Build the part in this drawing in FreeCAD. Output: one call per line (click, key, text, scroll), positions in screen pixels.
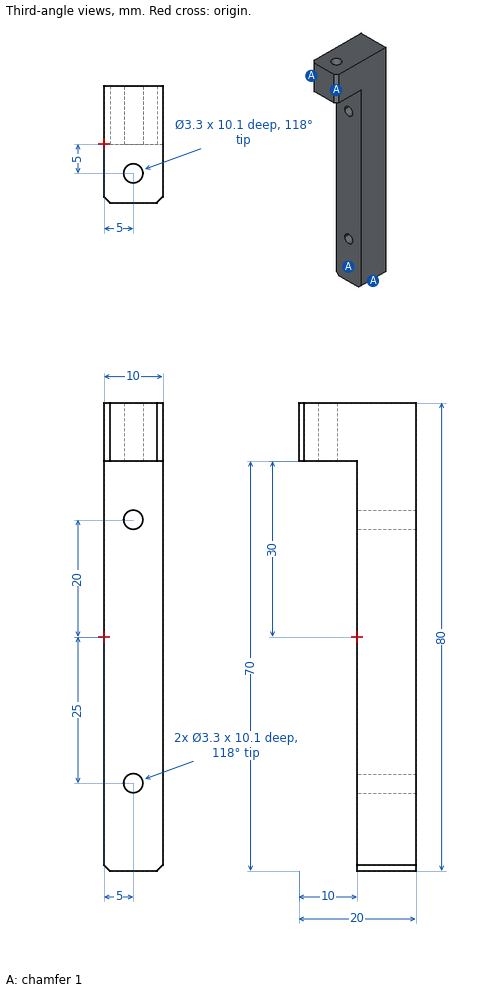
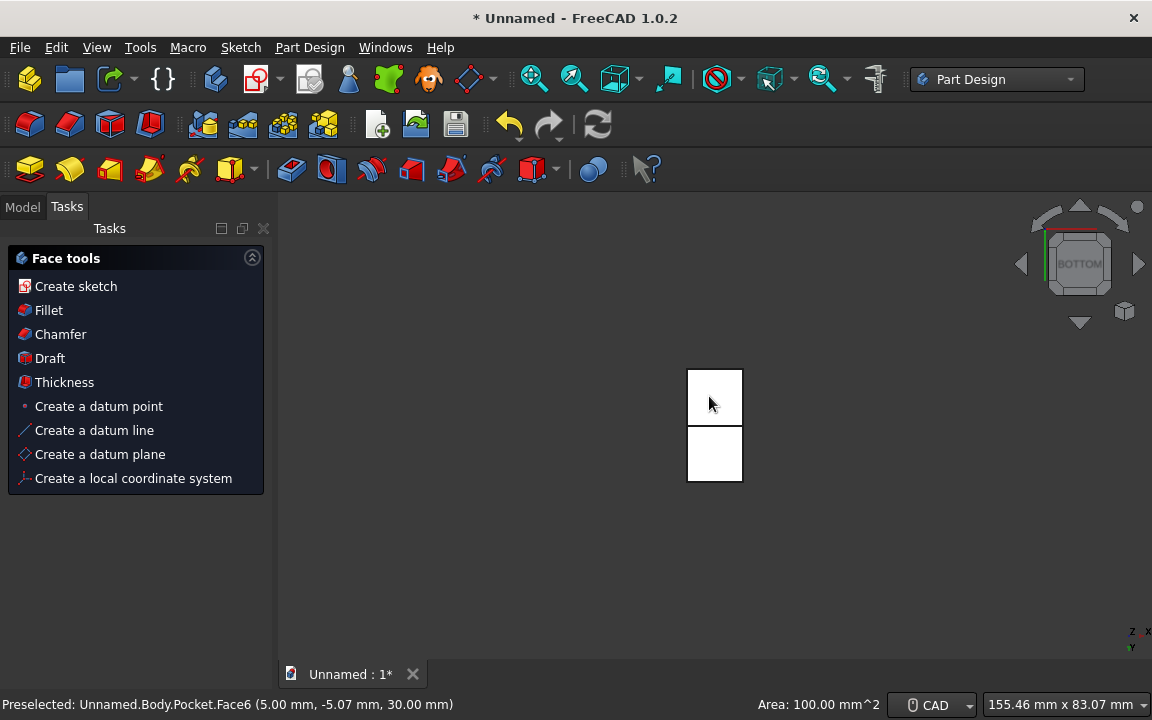
click(256, 80)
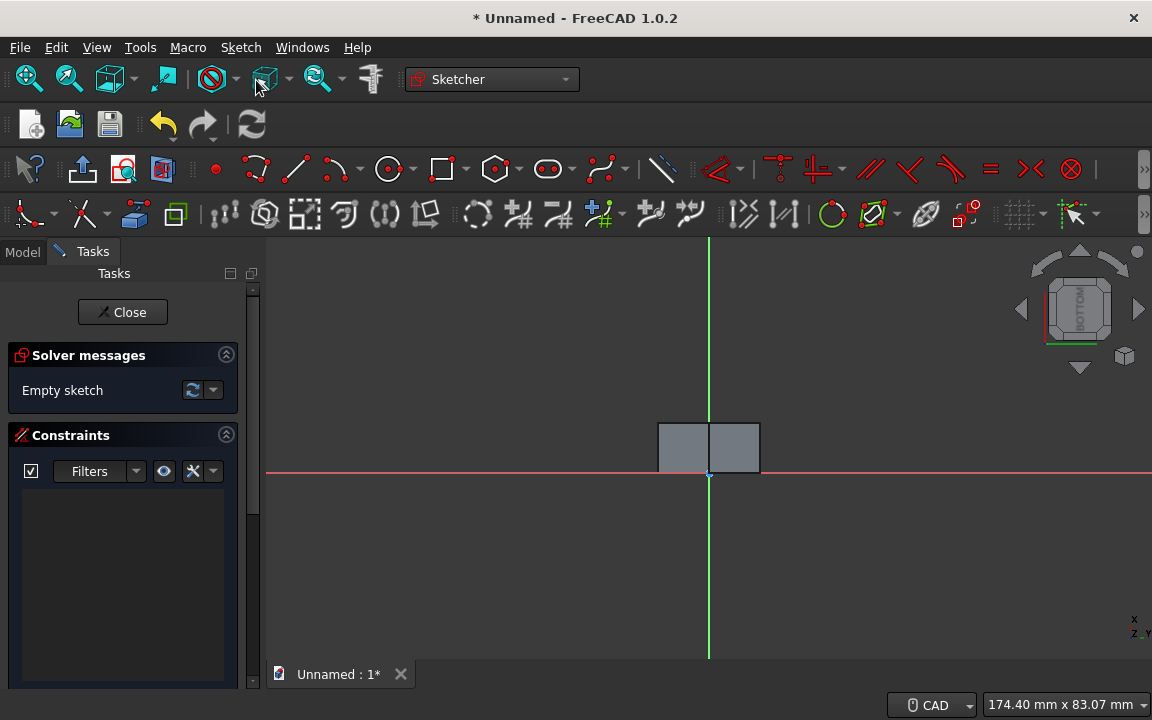
click(164, 170)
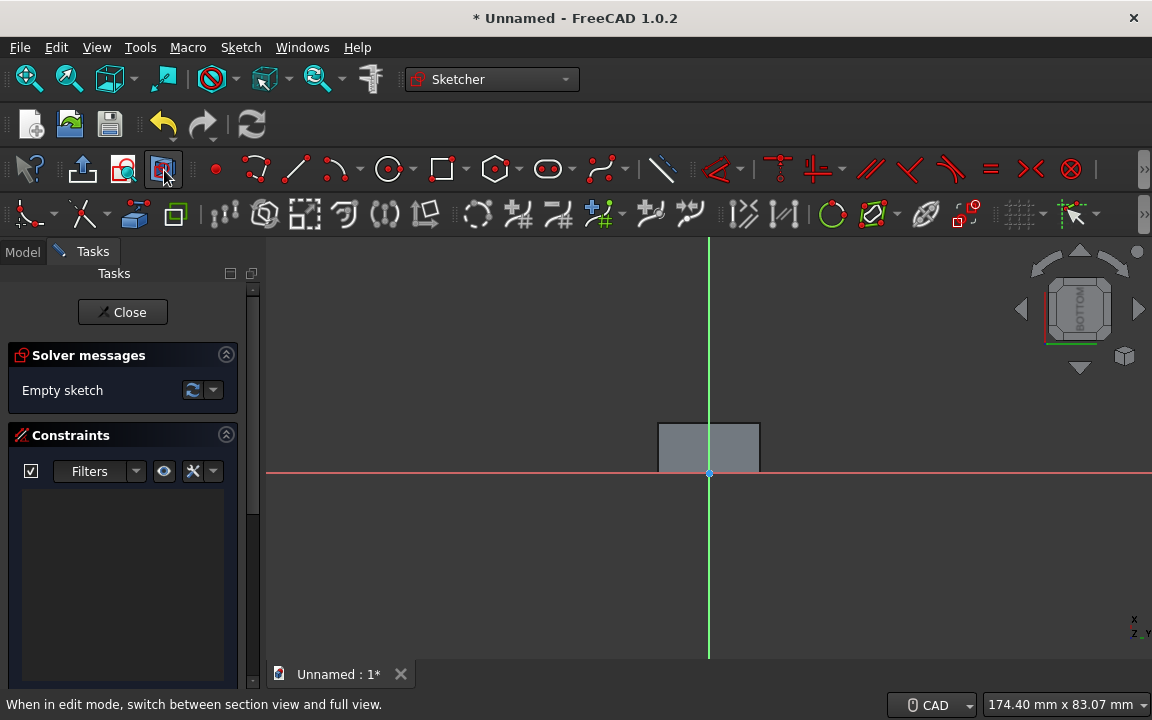
scroll(700, 458, up, 10)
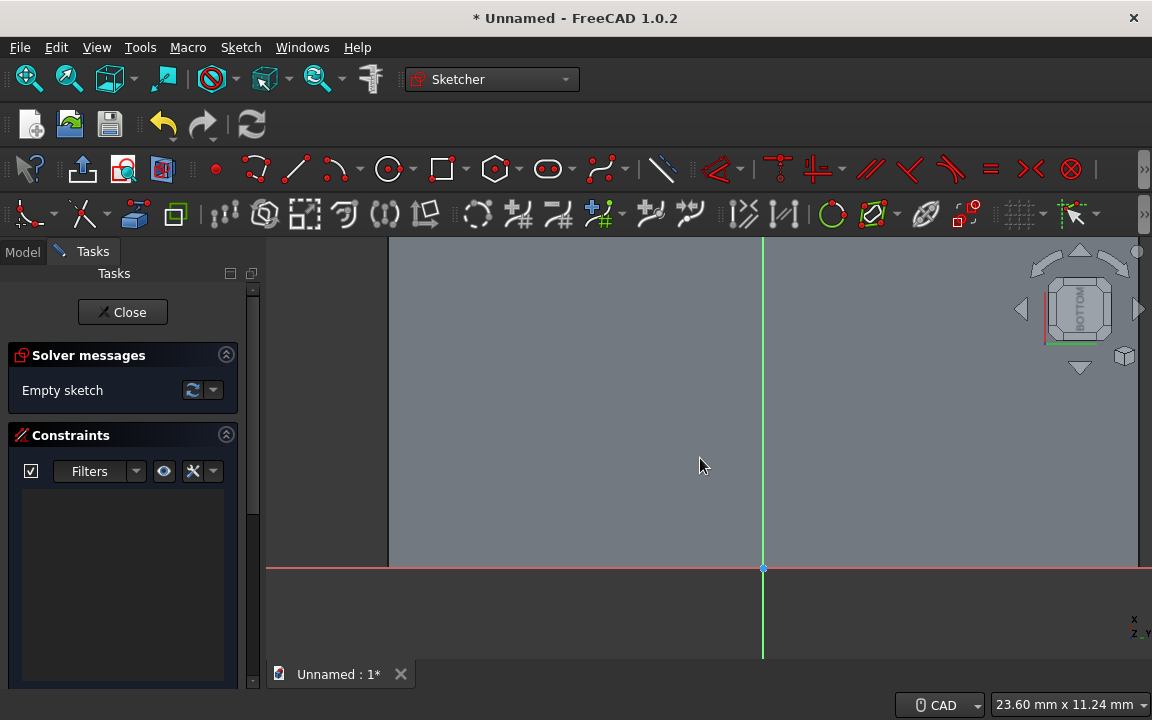
click(390, 170)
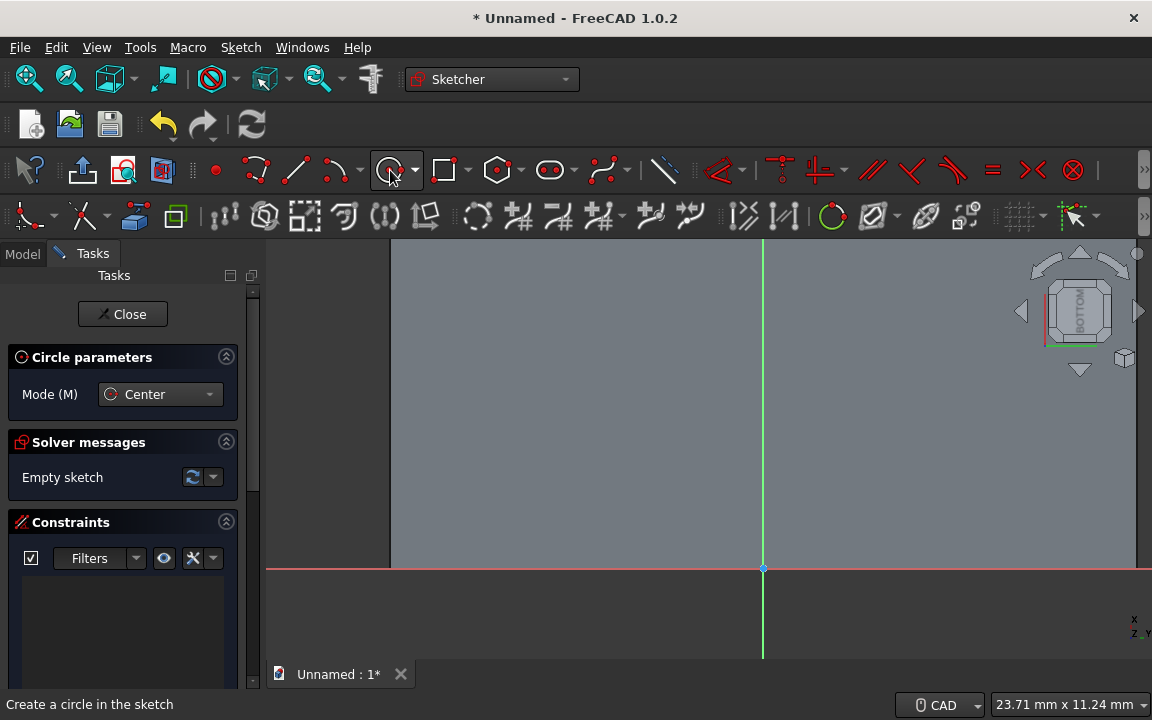
click(576, 382)
move(620, 338)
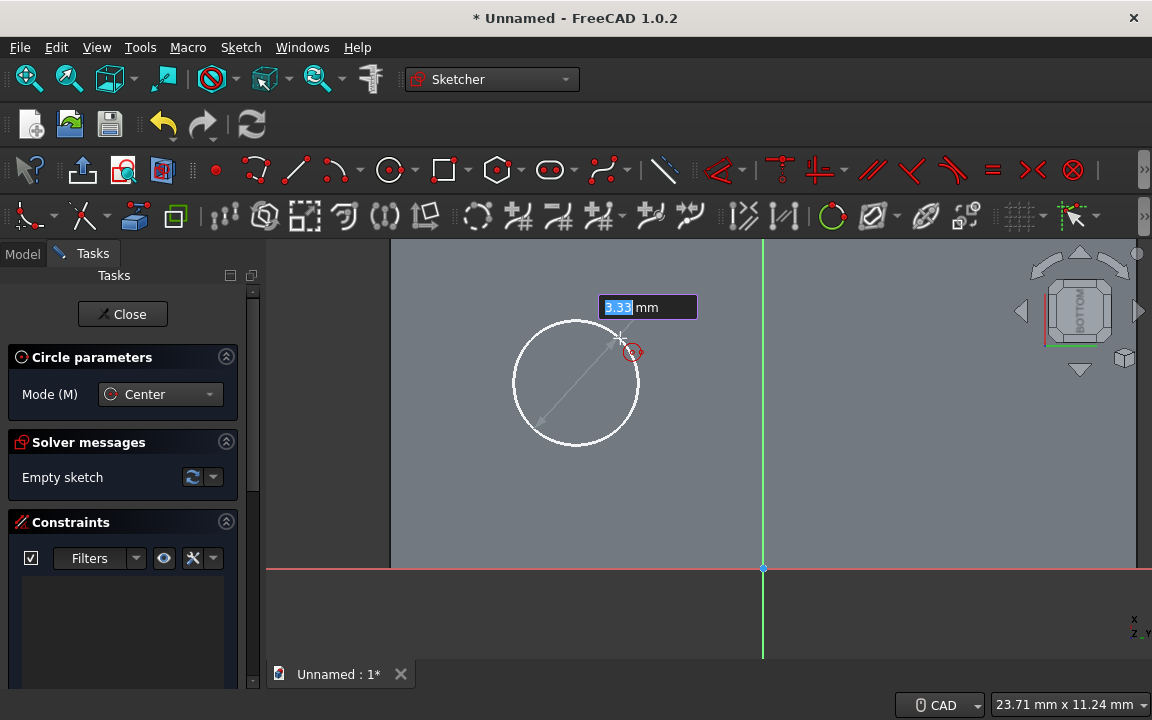
text(3.3)
key(Return)
key(Escape)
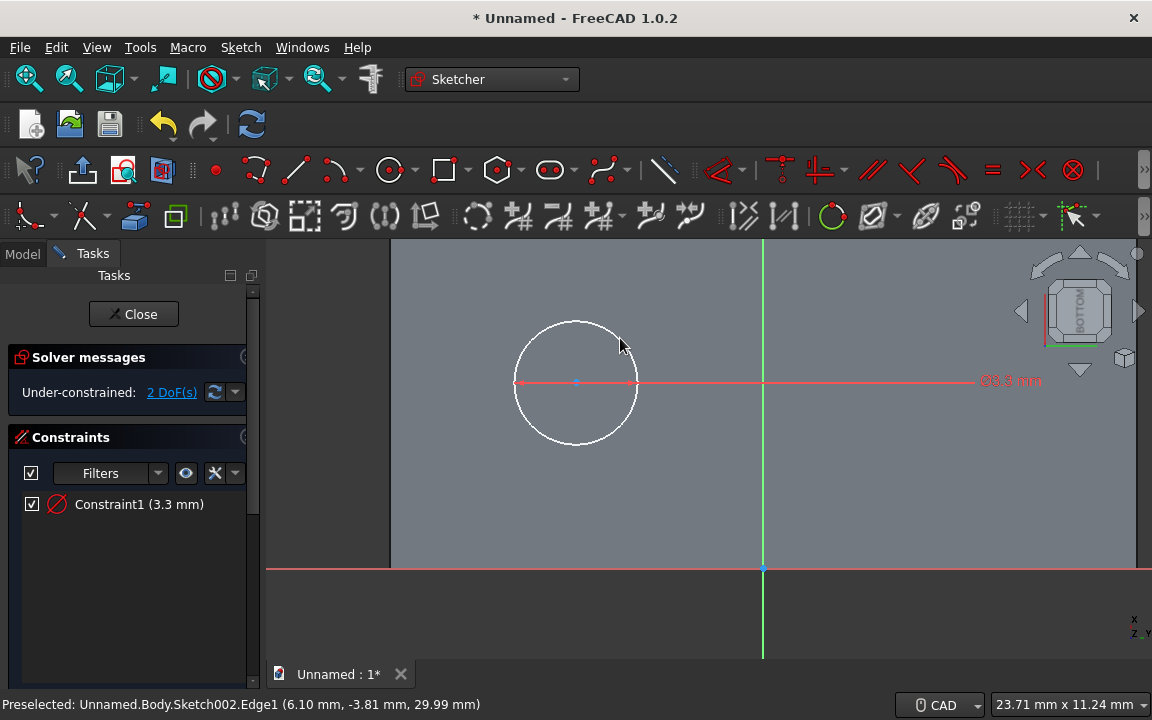
click(576, 383)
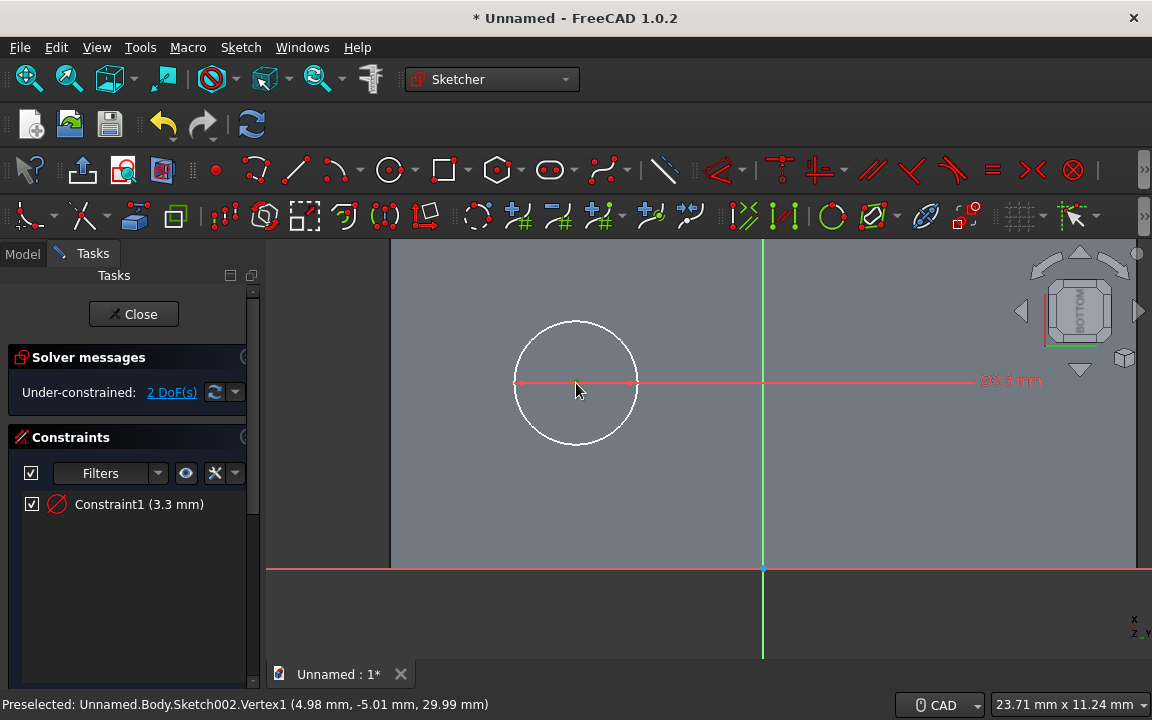
key(l)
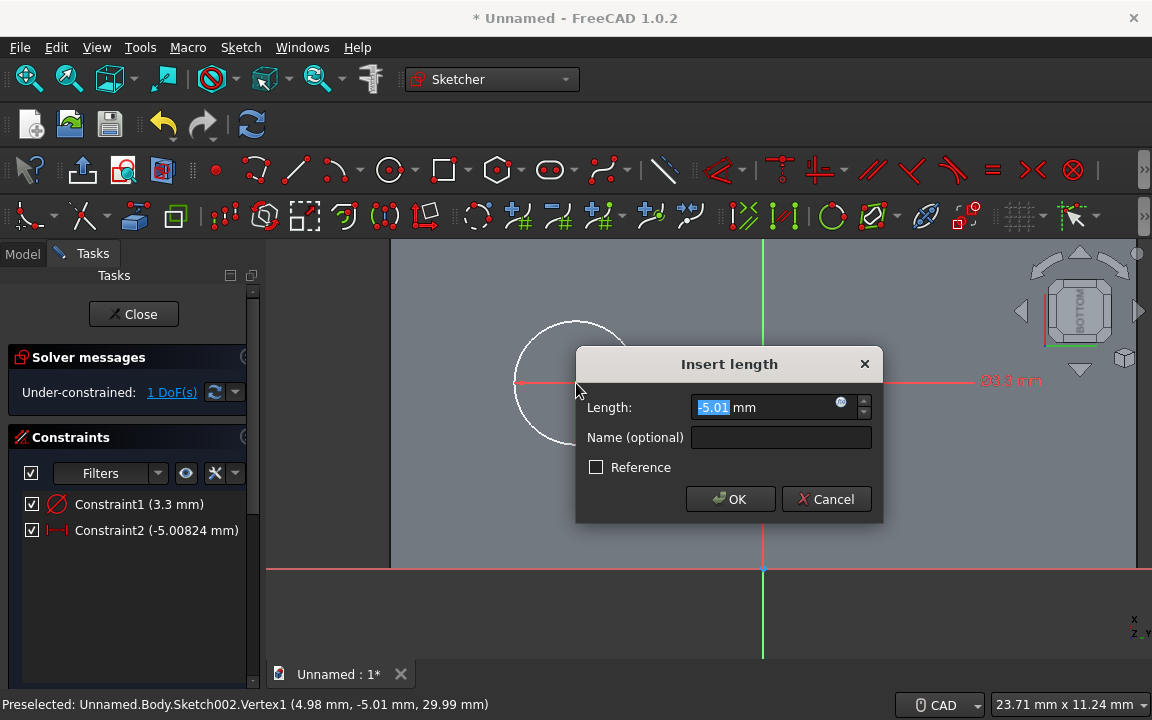
text(-5)
key(Return)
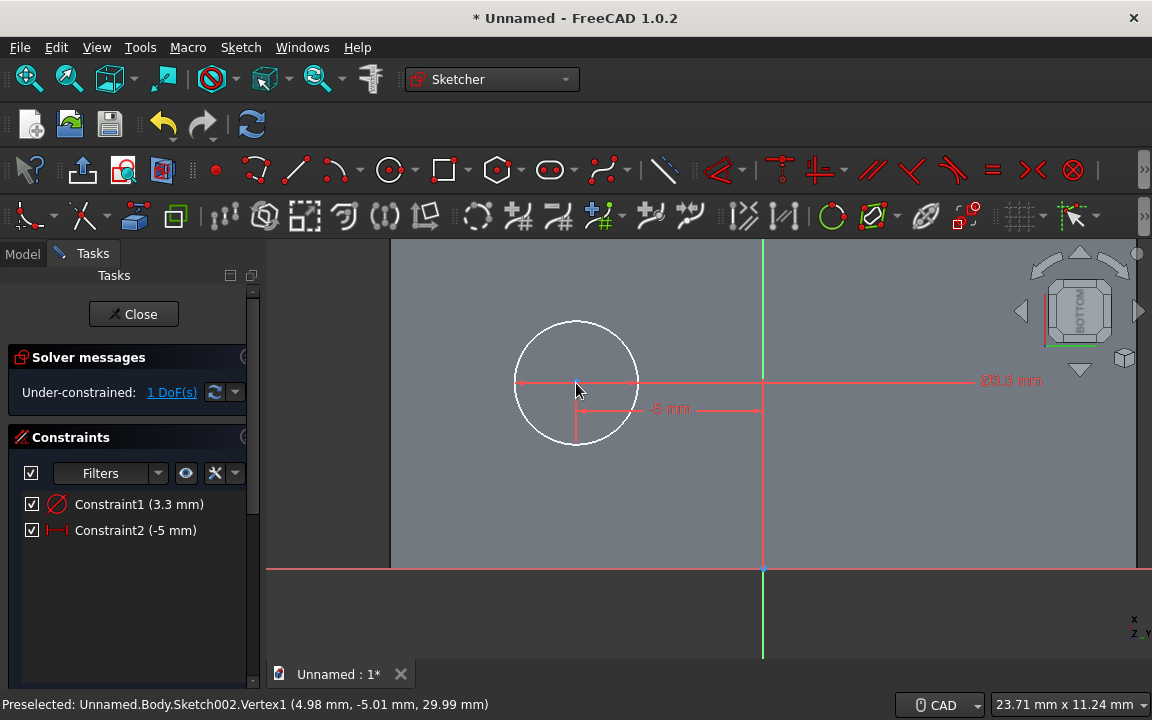
click(576, 383)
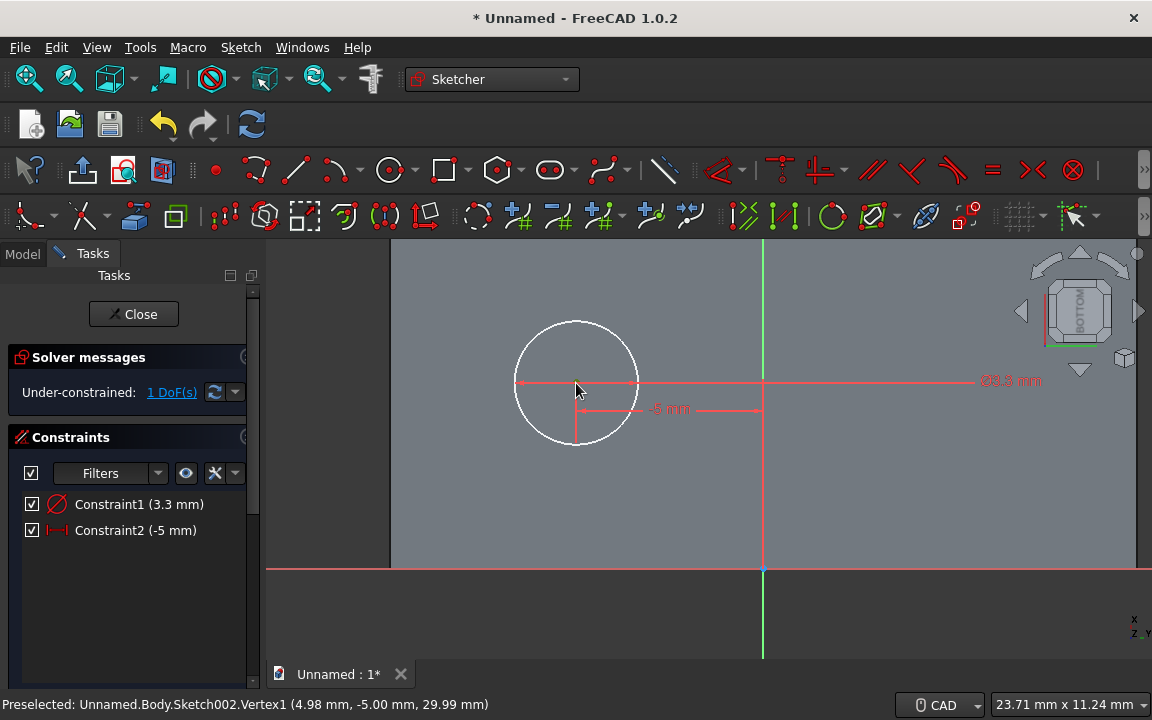
key(i)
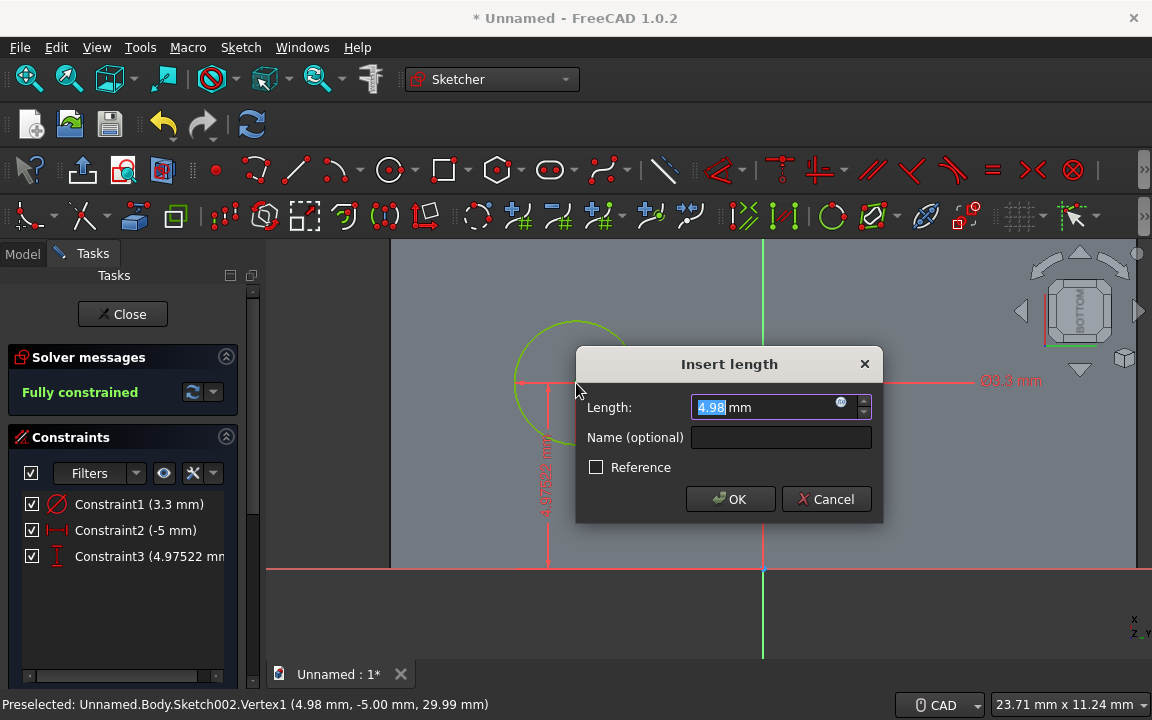
text(5)
key(Return)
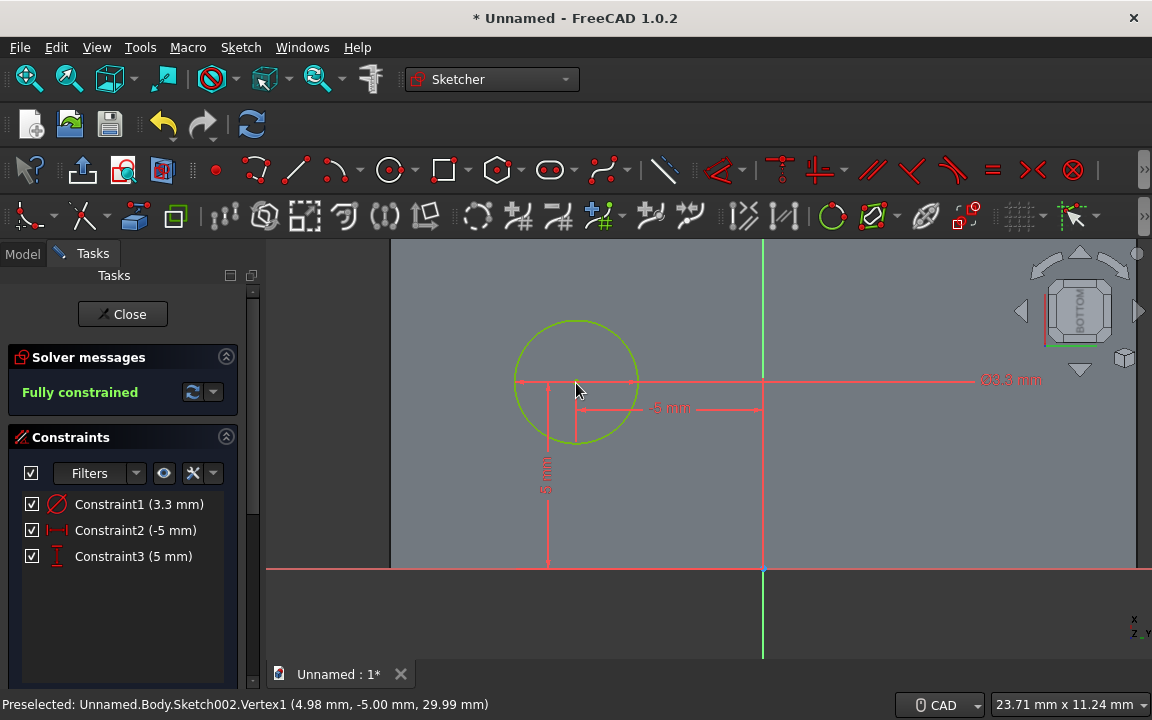
click(123, 314)